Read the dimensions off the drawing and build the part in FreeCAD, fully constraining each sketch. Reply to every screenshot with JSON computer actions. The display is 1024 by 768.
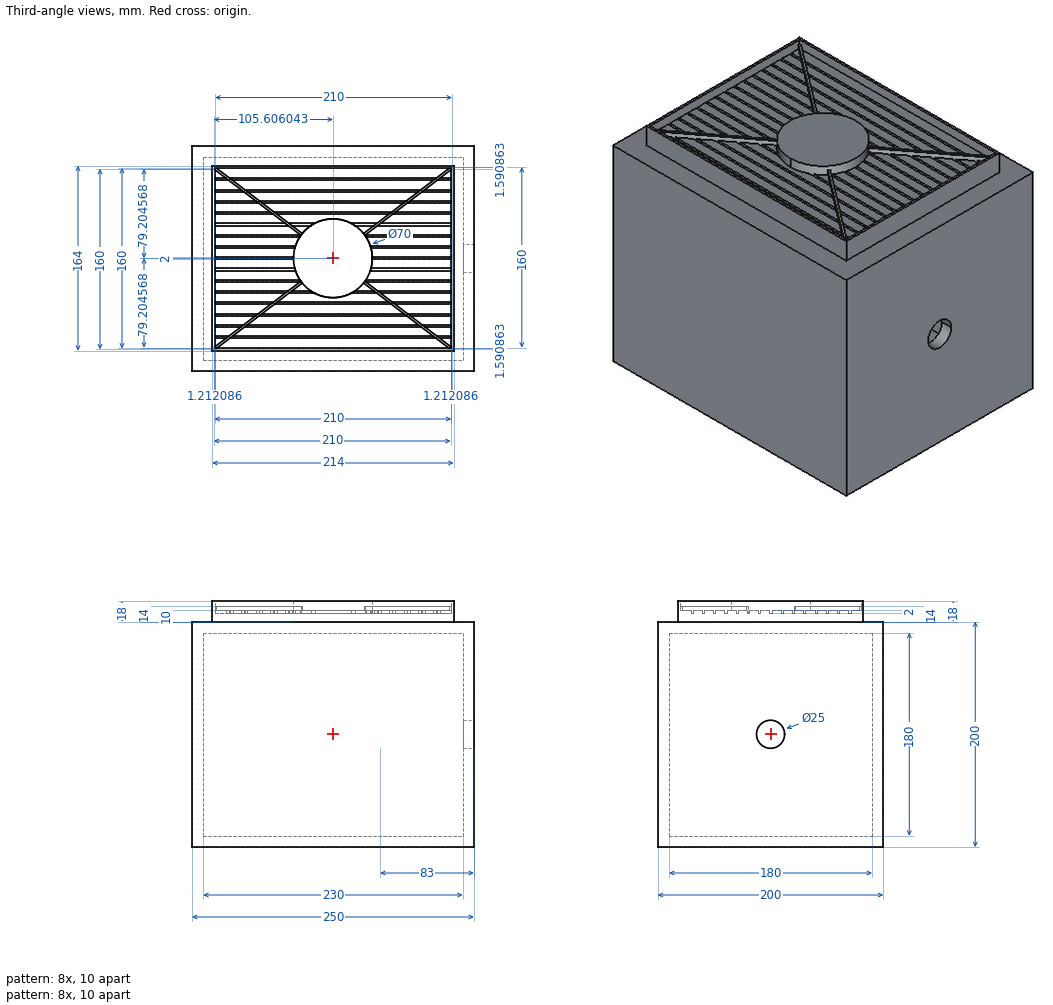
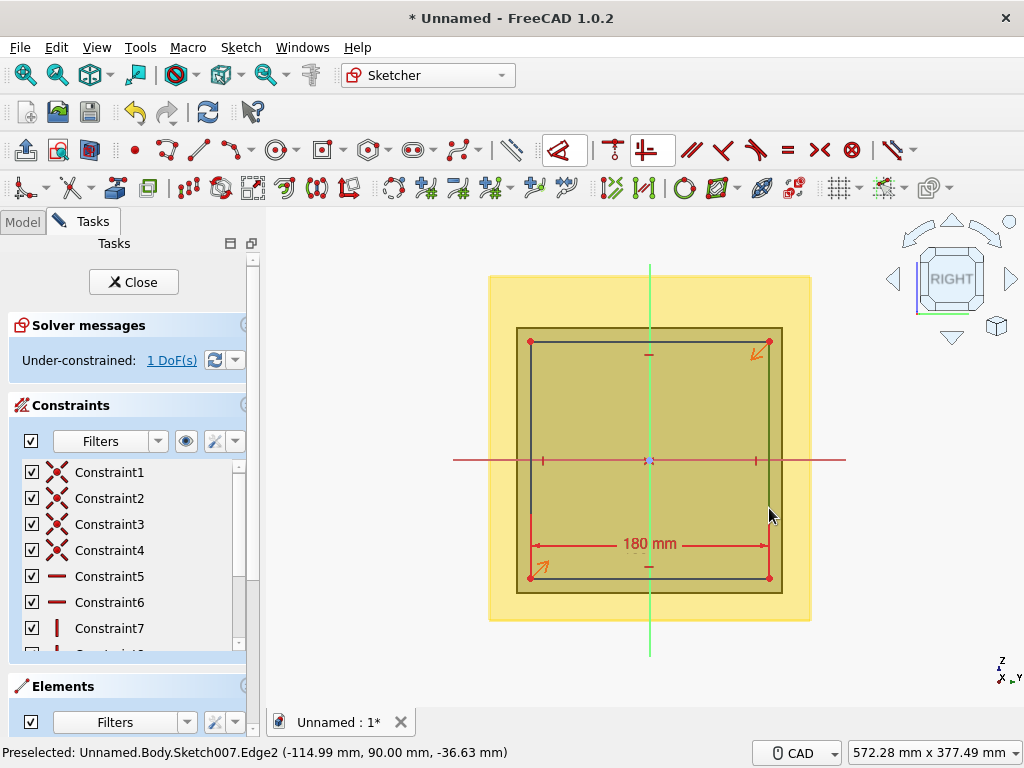
{"action": "left_click", "coordinate": [582, 150]}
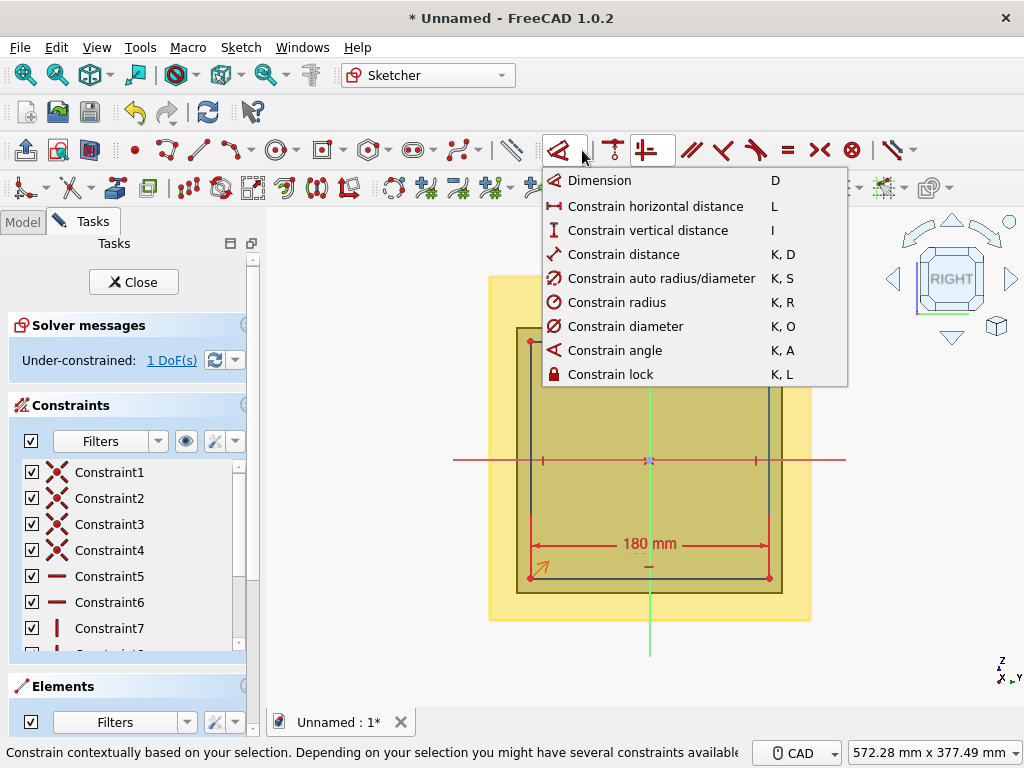
{"action": "left_click", "coordinate": [695, 230]}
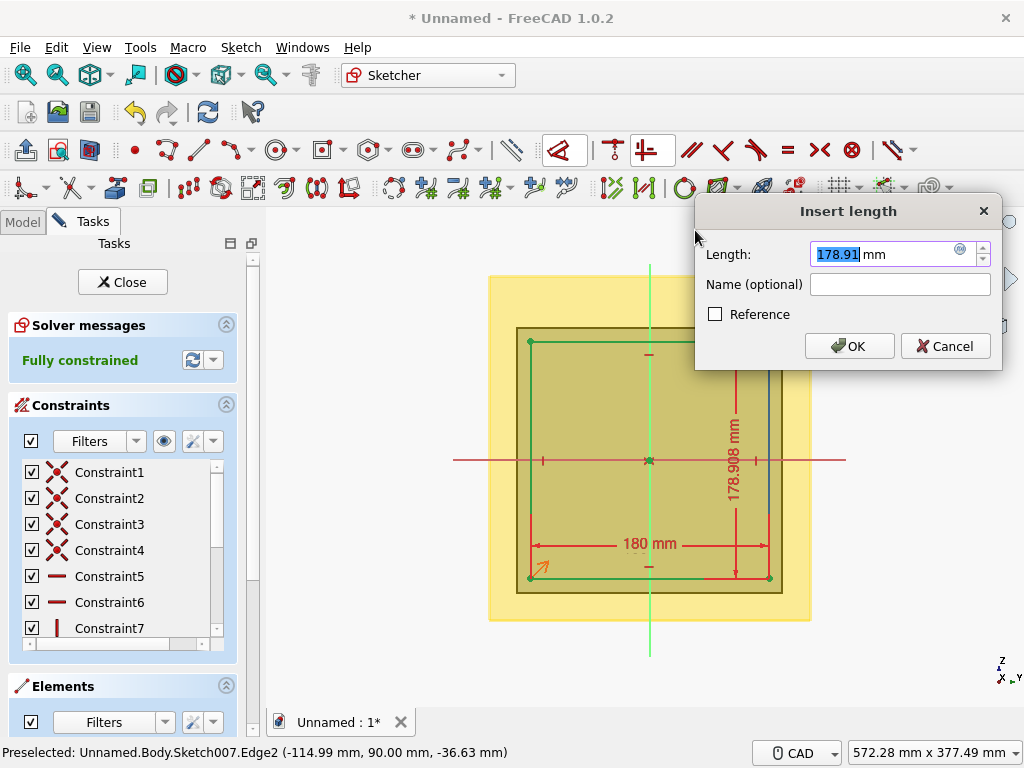
{"action": "type", "text": "180"}
{"action": "key", "text": "Return"}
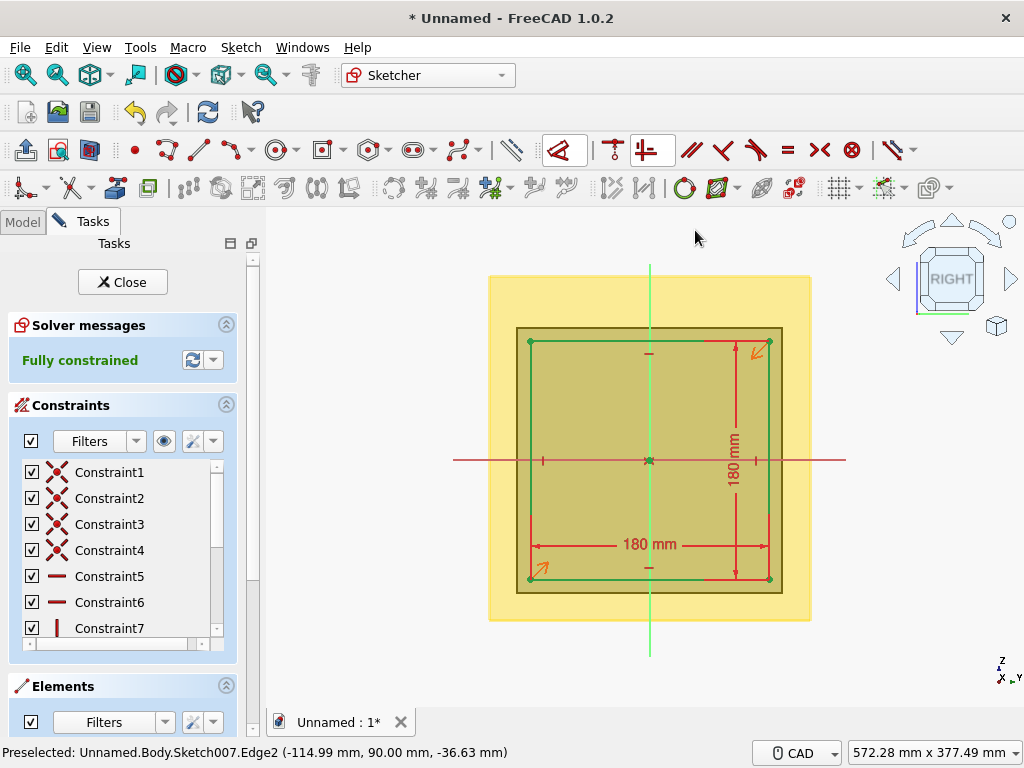
{"action": "left_click", "coordinate": [123, 282]}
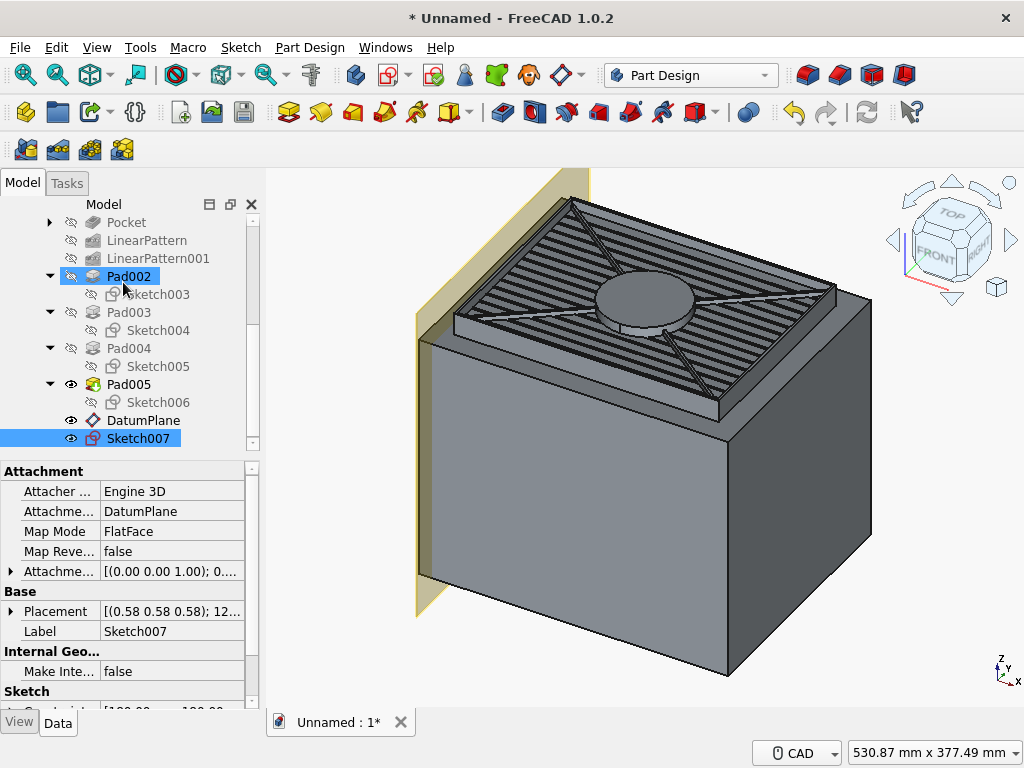
{"action": "left_click", "coordinate": [504, 112]}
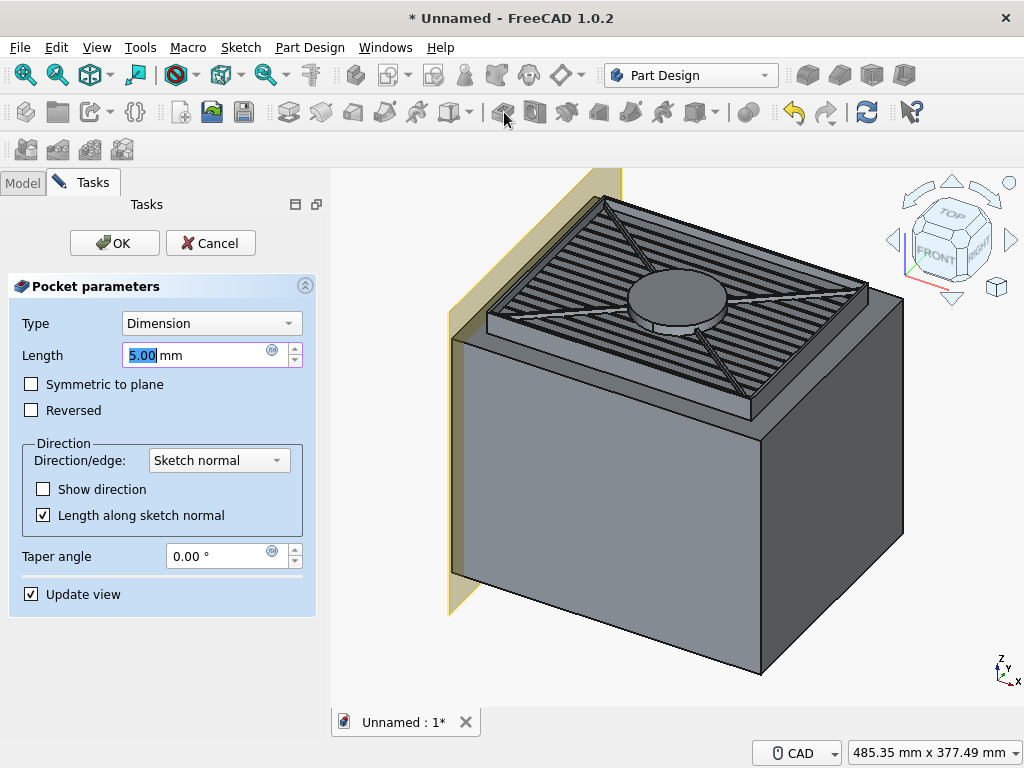
{"action": "type", "text": "230"}
{"action": "key", "text": "Tab"}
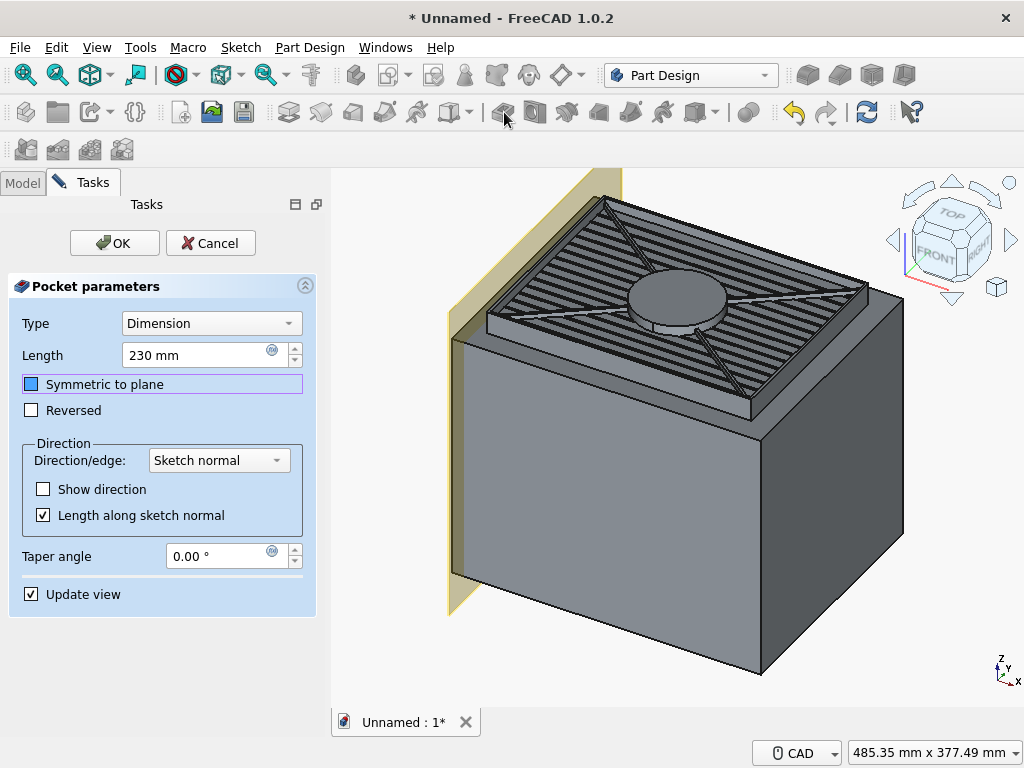
{"action": "left_click", "coordinate": [30, 410]}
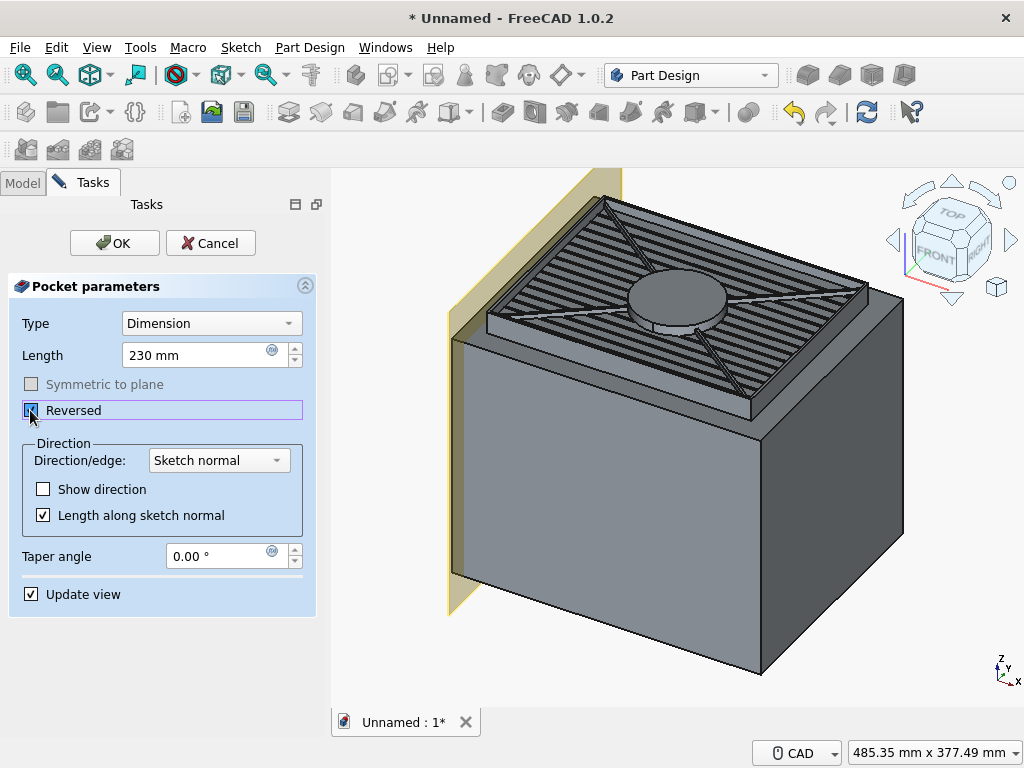
{"action": "left_click", "coordinate": [115, 243]}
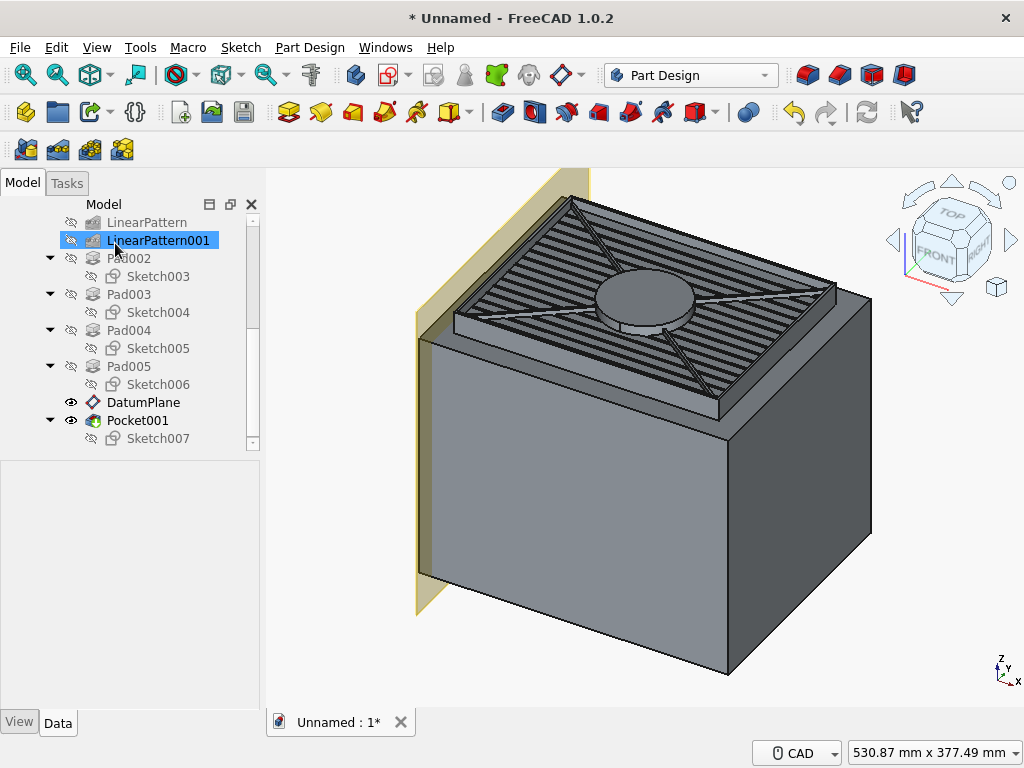
{"action": "left_click", "coordinate": [116, 402]}
{"action": "key", "text": "space"}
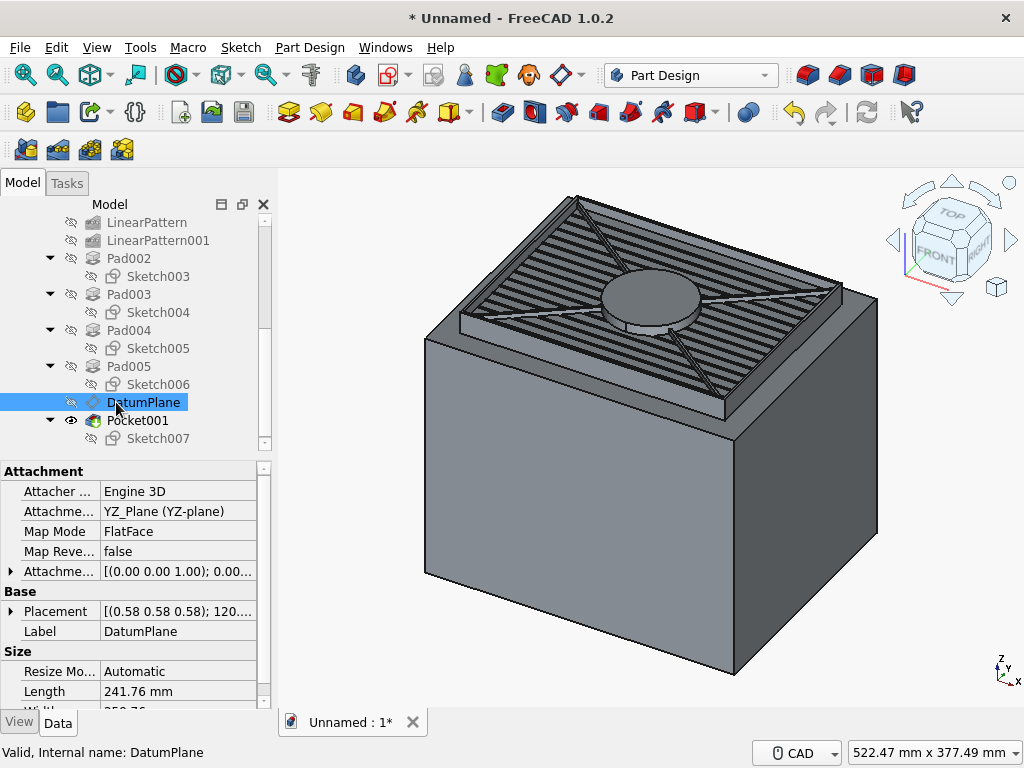
{"action": "left_click", "coordinate": [806, 486]}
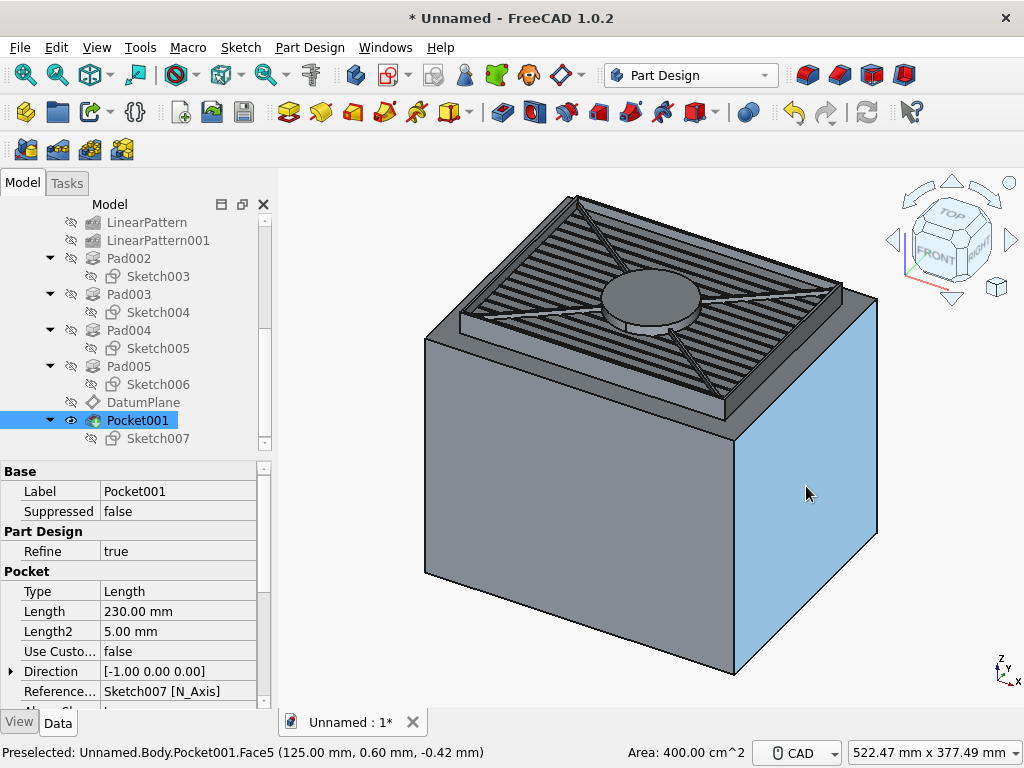
{"action": "left_click", "coordinate": [388, 76]}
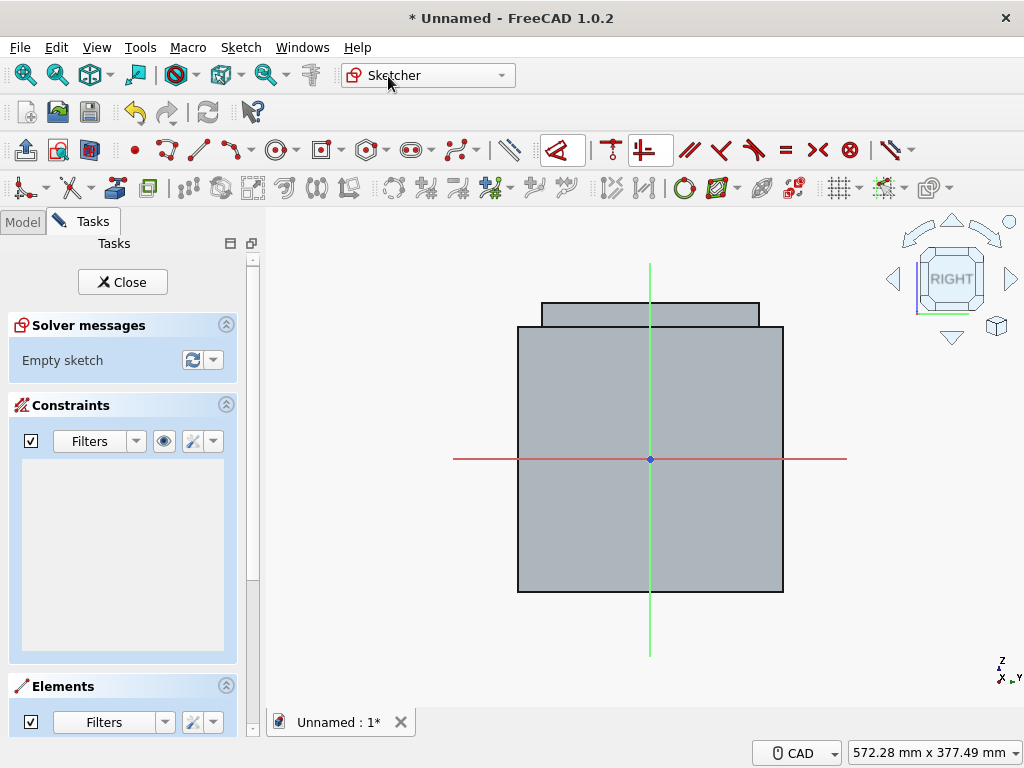
{"action": "scroll", "coordinate": [660, 460], "scroll_direction": "up", "scroll_amount": 11}